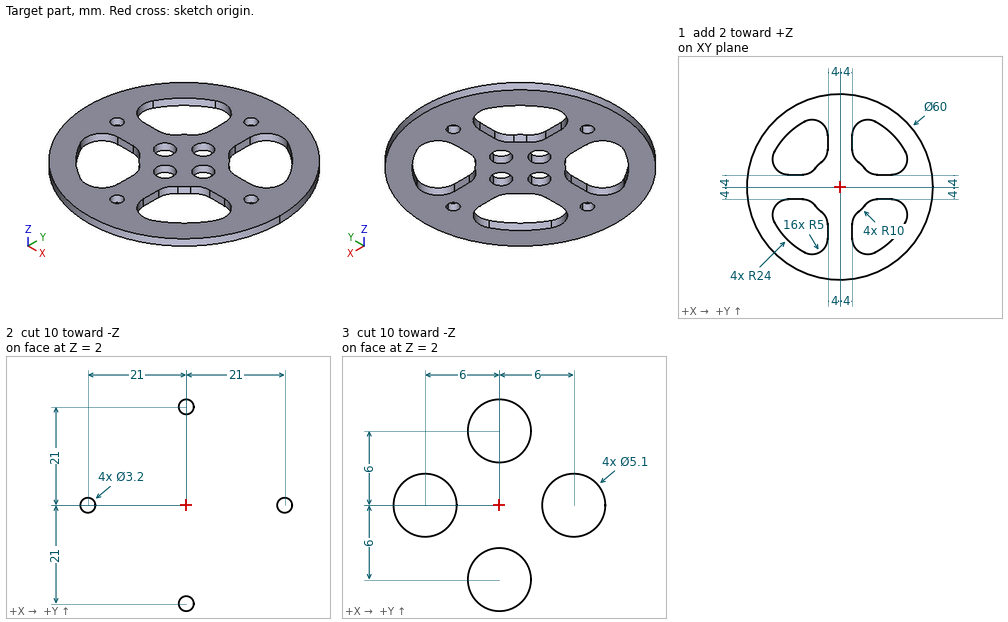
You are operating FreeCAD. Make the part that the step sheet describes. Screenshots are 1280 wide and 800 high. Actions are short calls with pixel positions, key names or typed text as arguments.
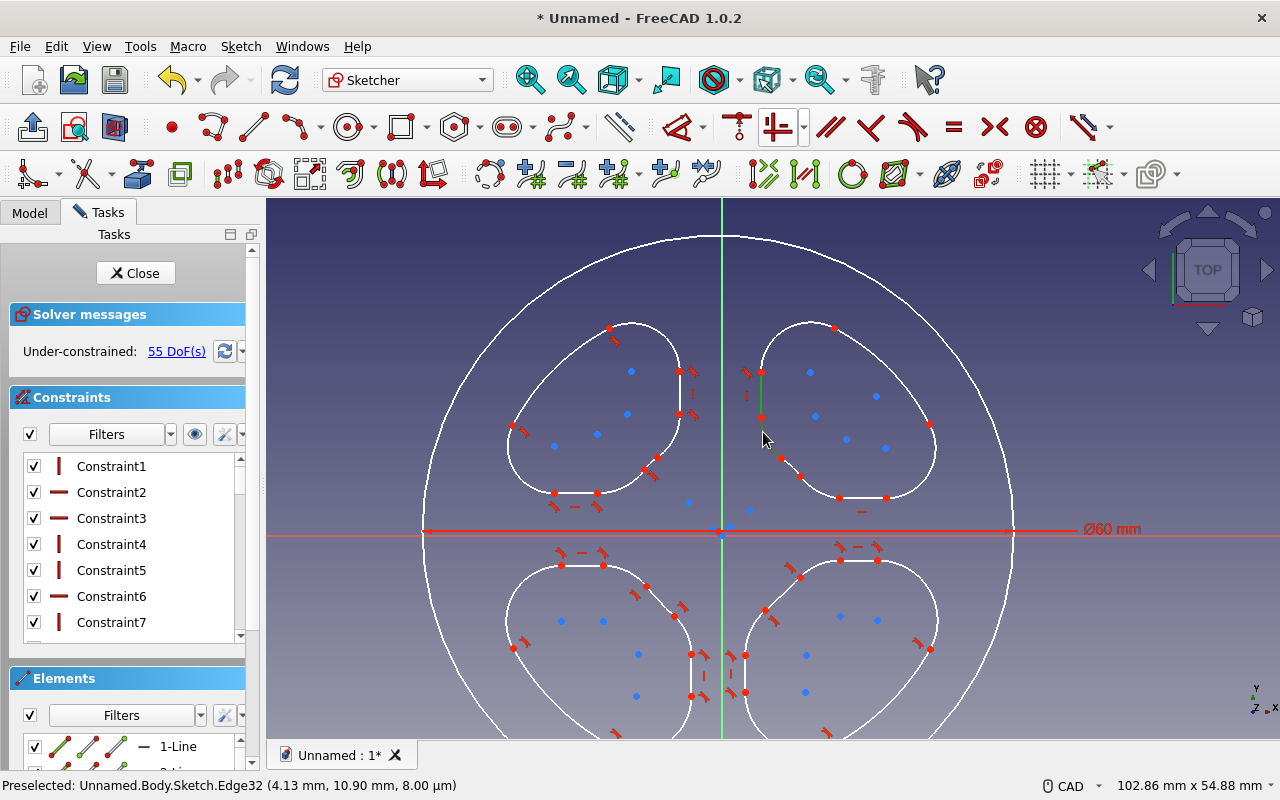
click(913, 128)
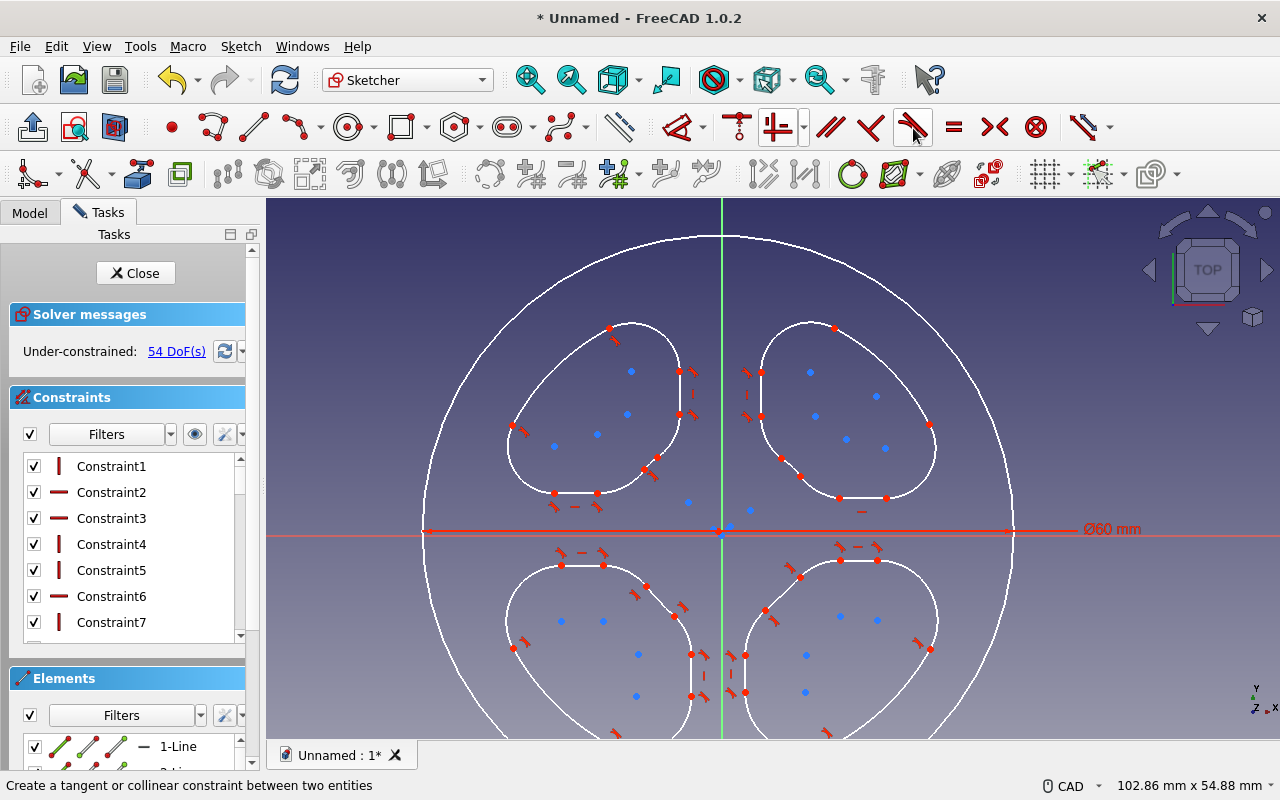
click(872, 498)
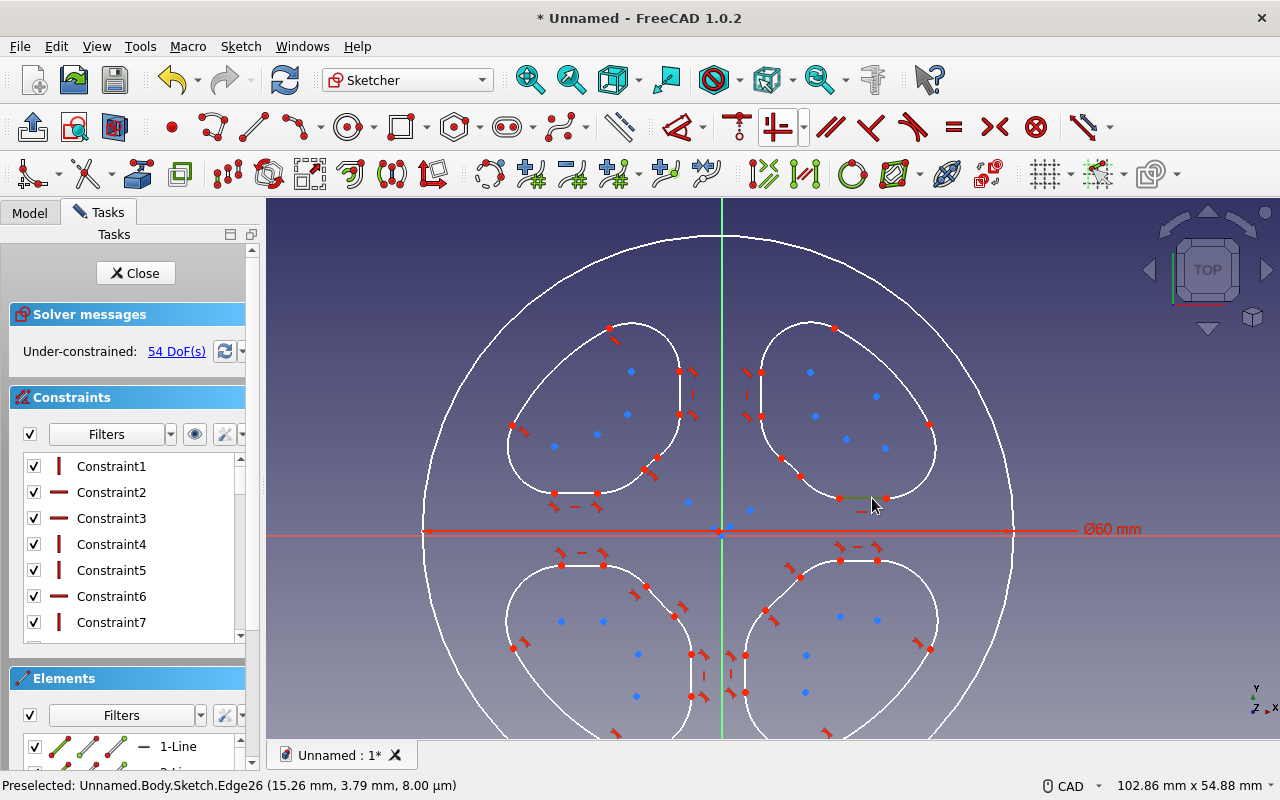
click(915, 489)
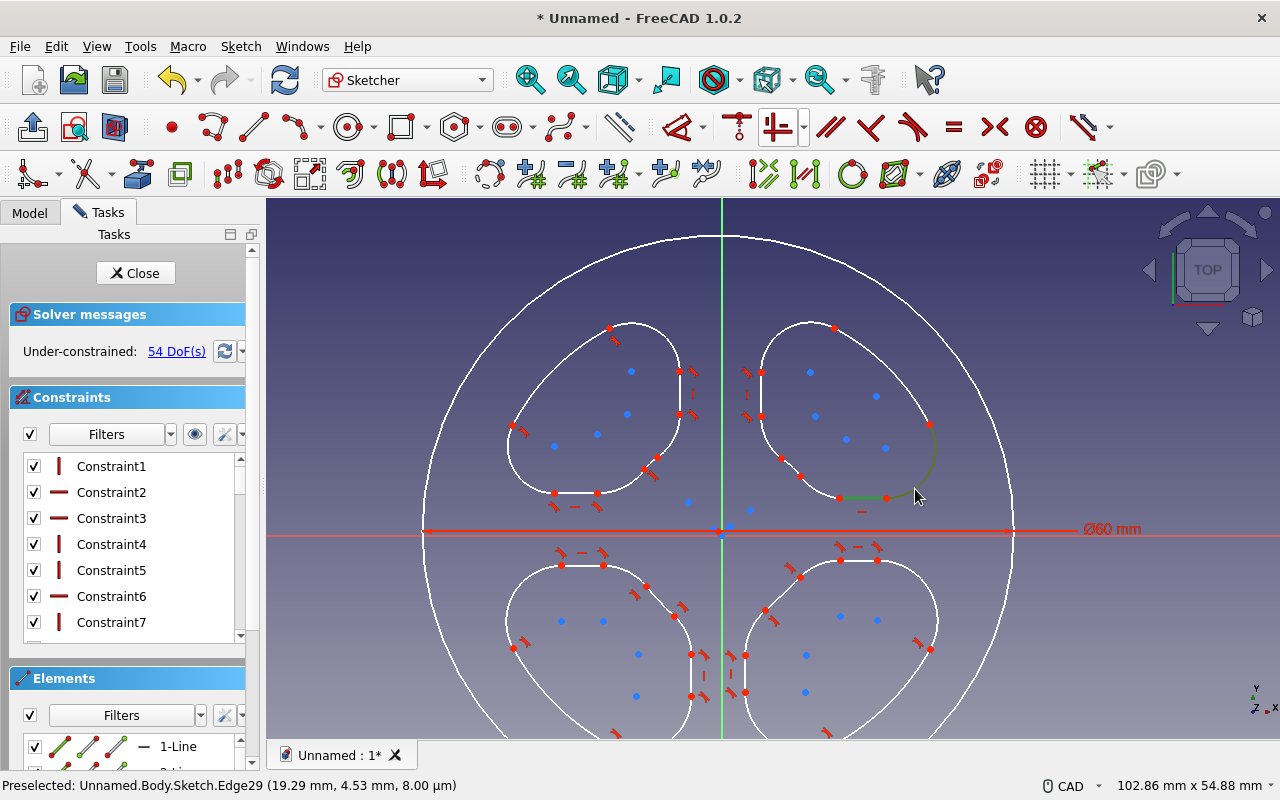
key(t)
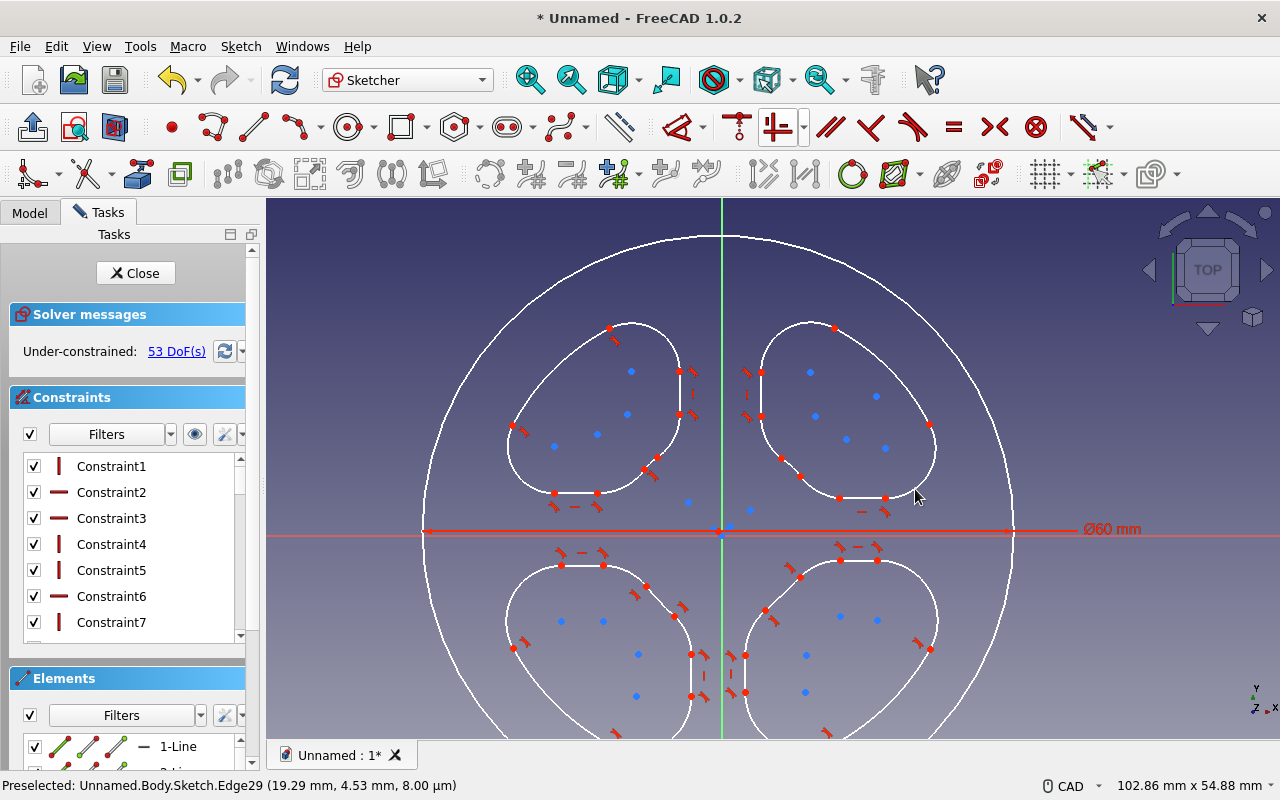
click(872, 498)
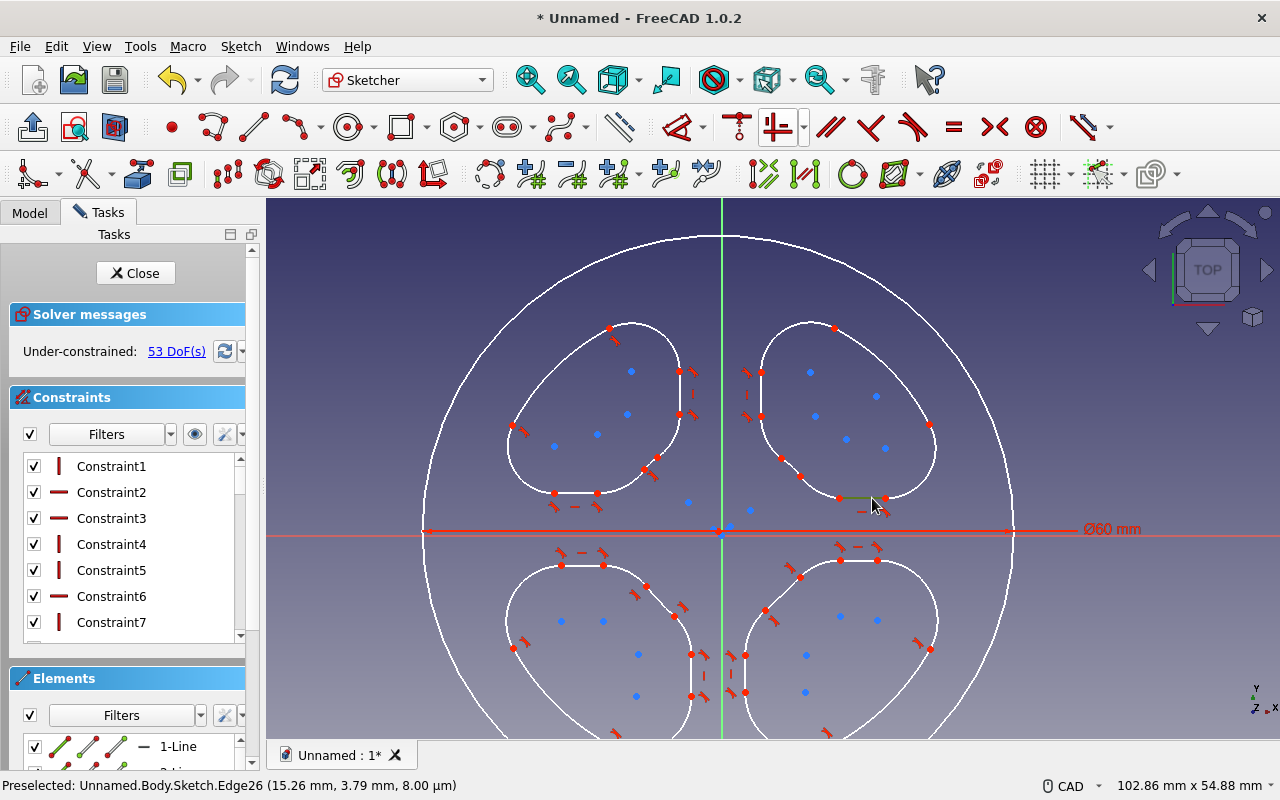
click(810, 486)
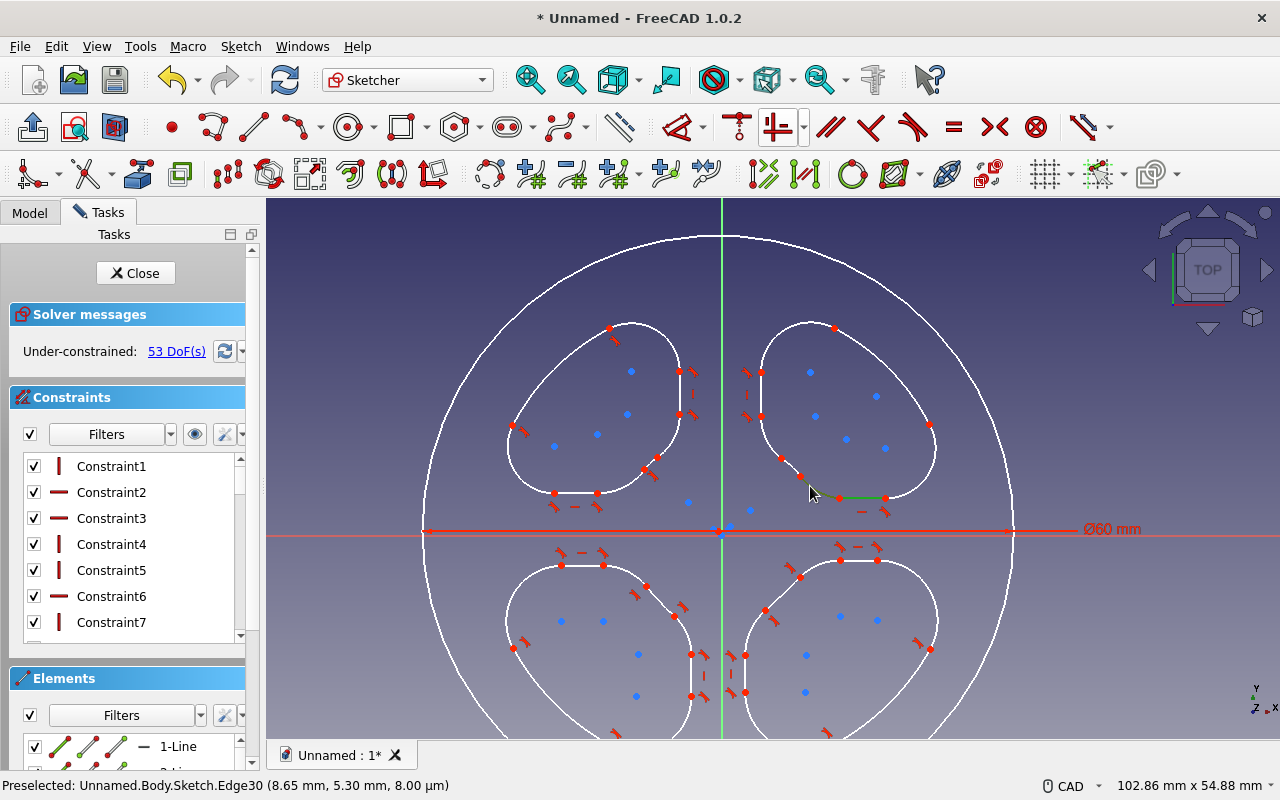
click(913, 128)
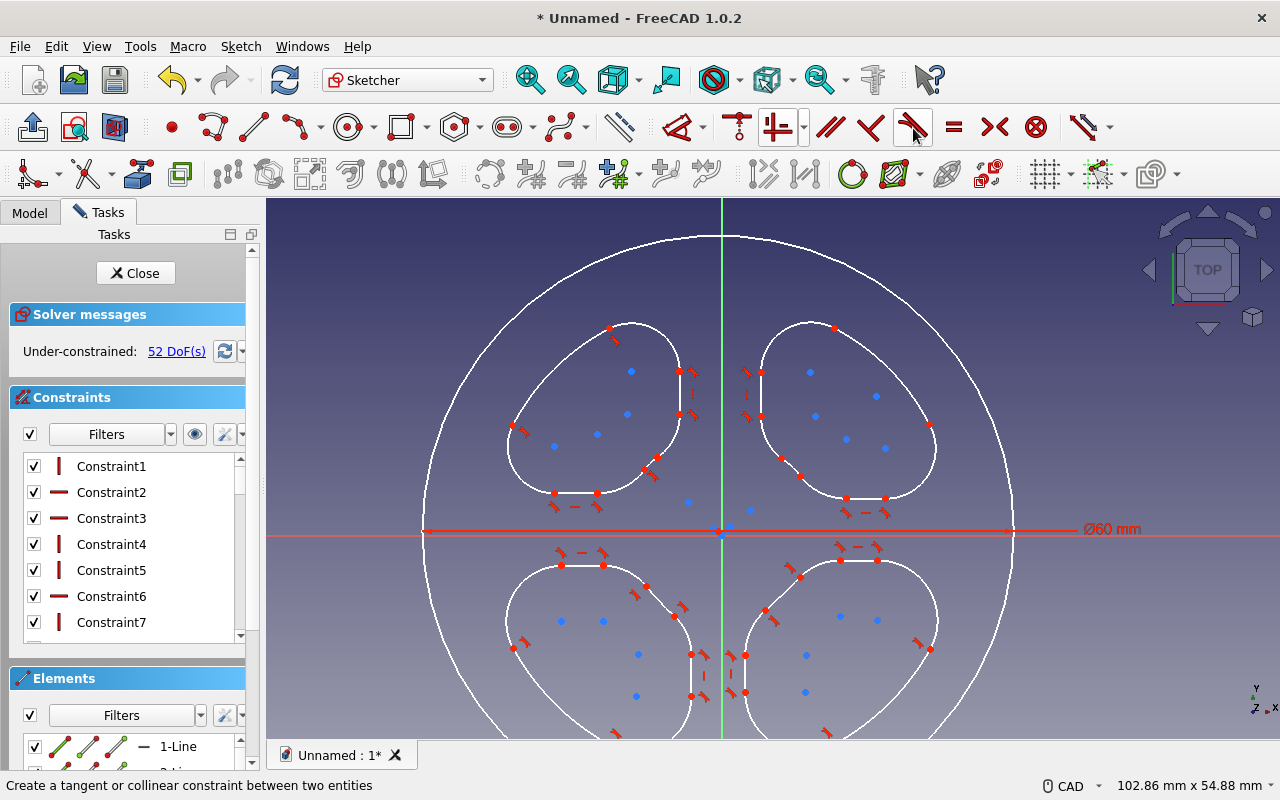
click(804, 323)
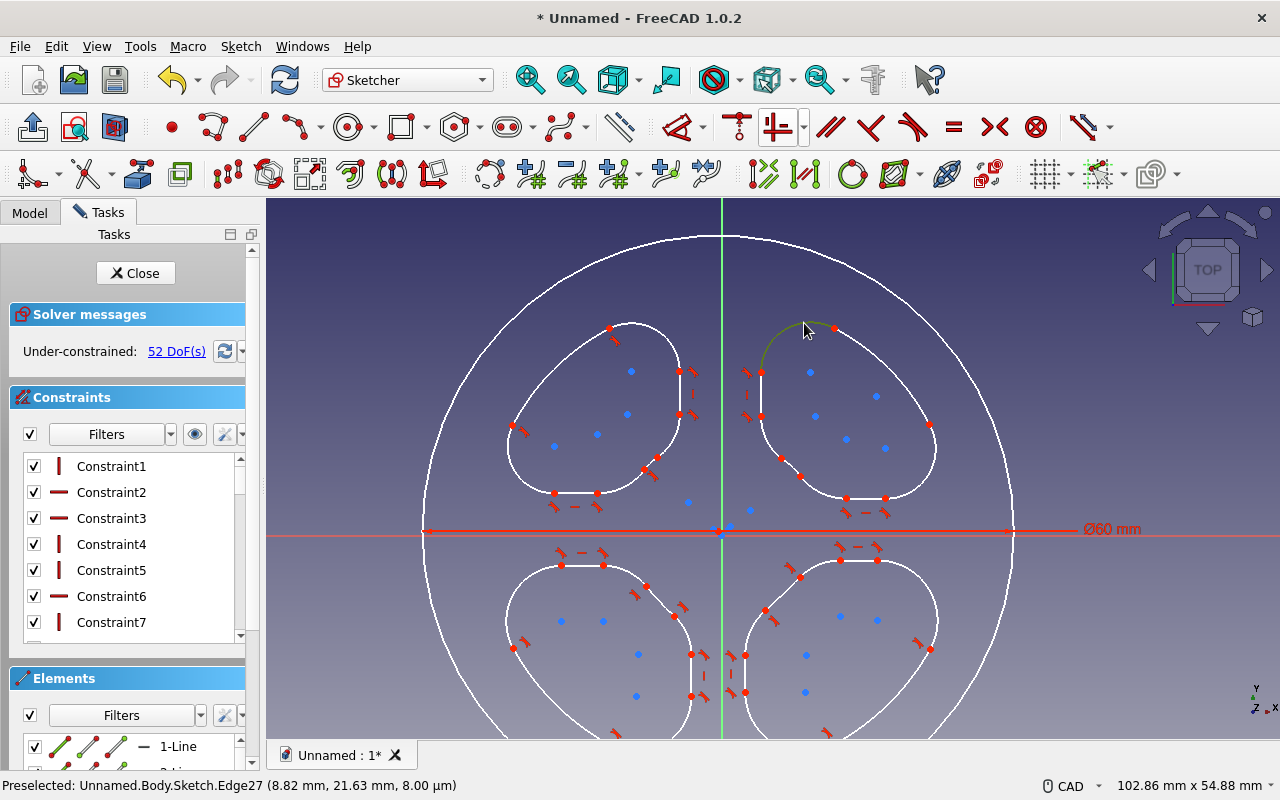
click(908, 390)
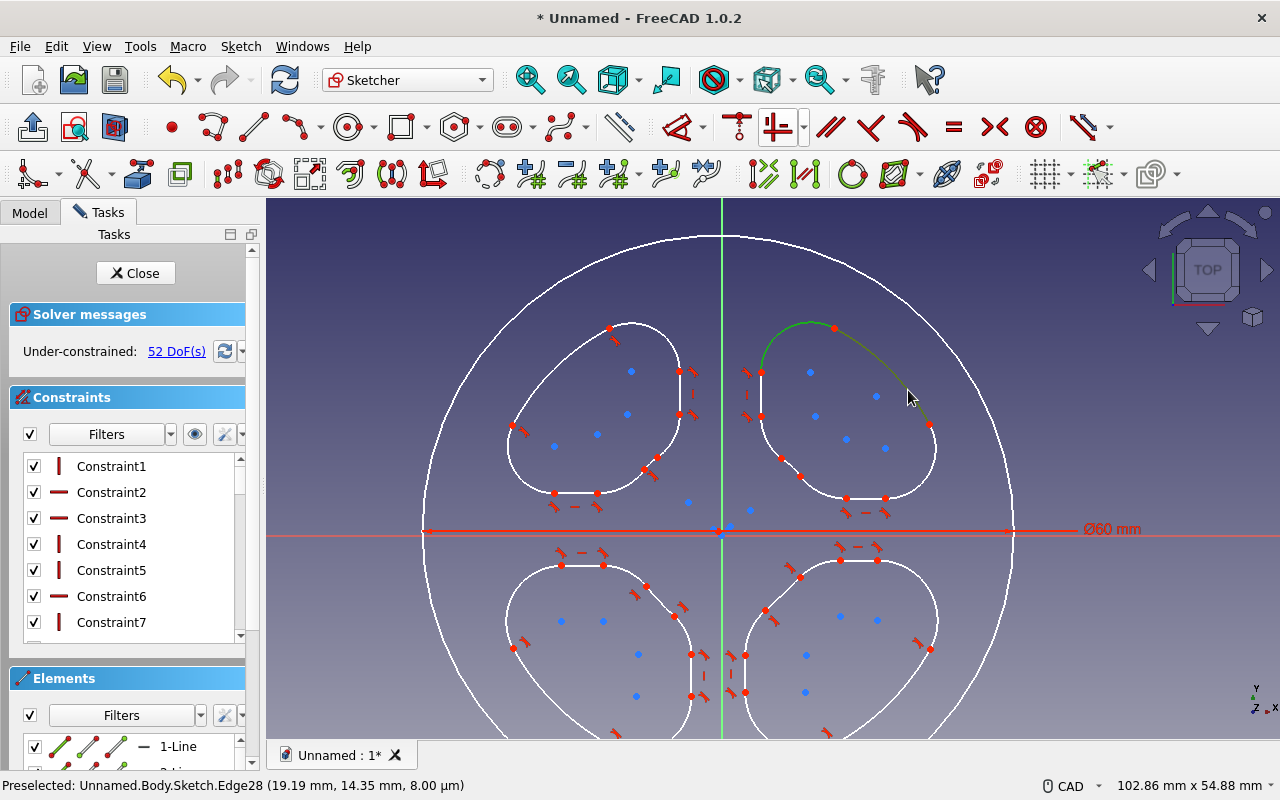
click(913, 128)